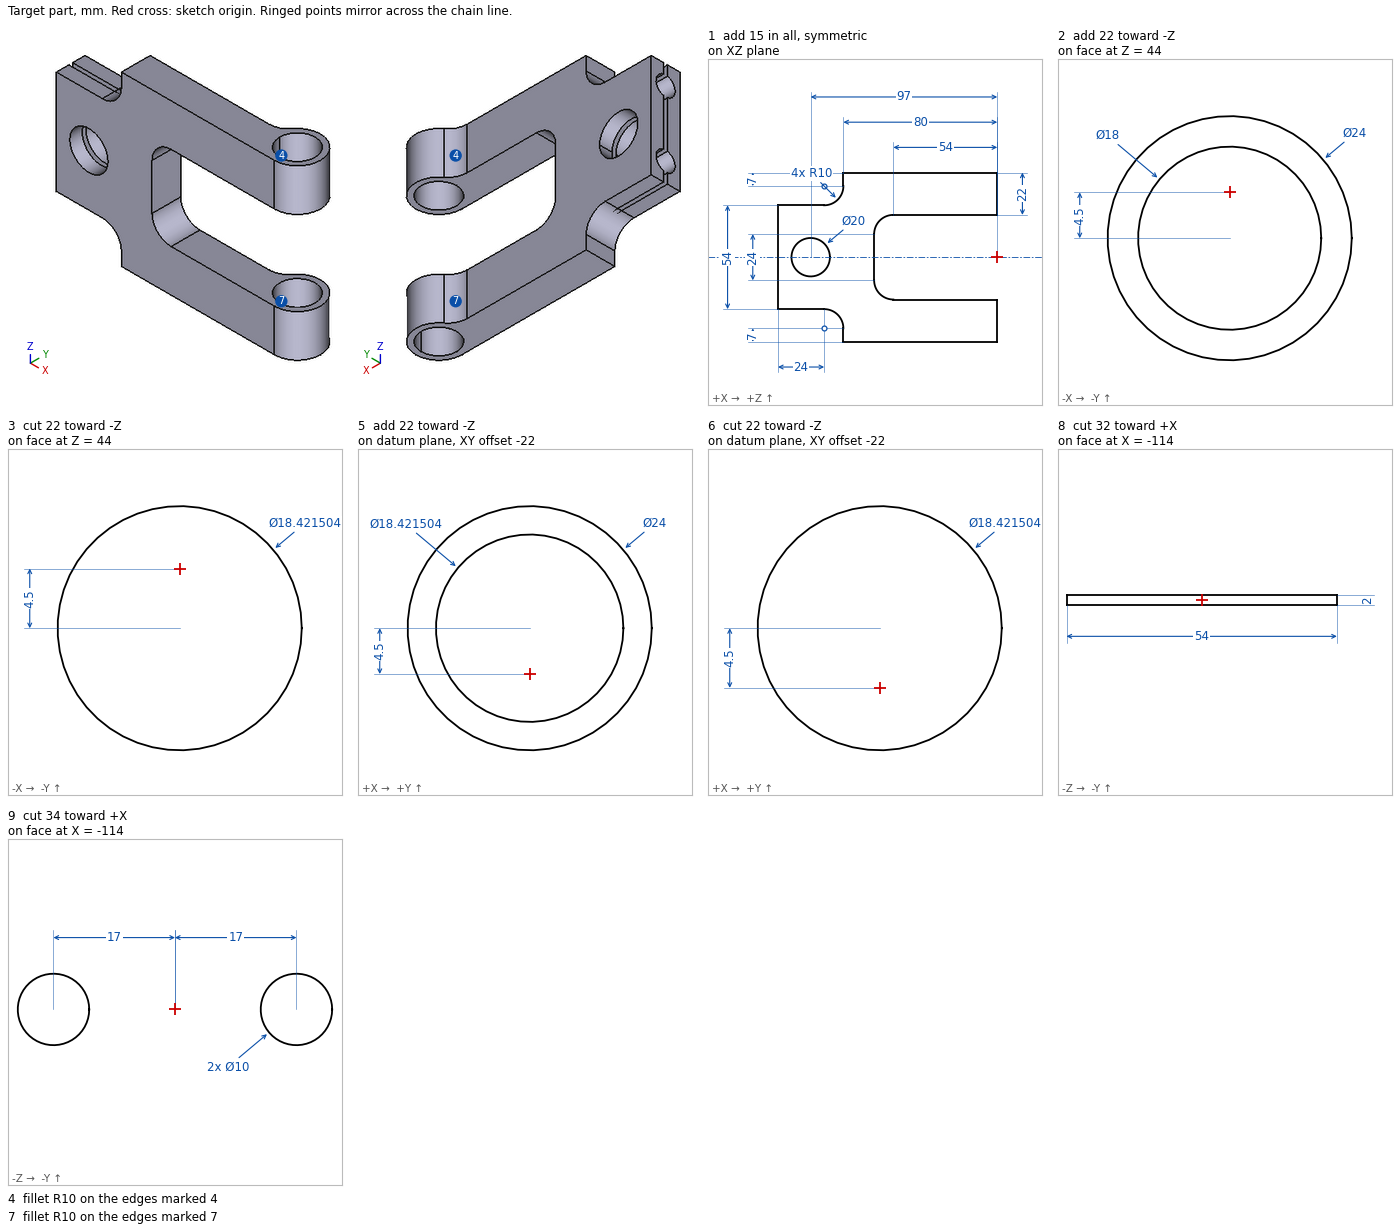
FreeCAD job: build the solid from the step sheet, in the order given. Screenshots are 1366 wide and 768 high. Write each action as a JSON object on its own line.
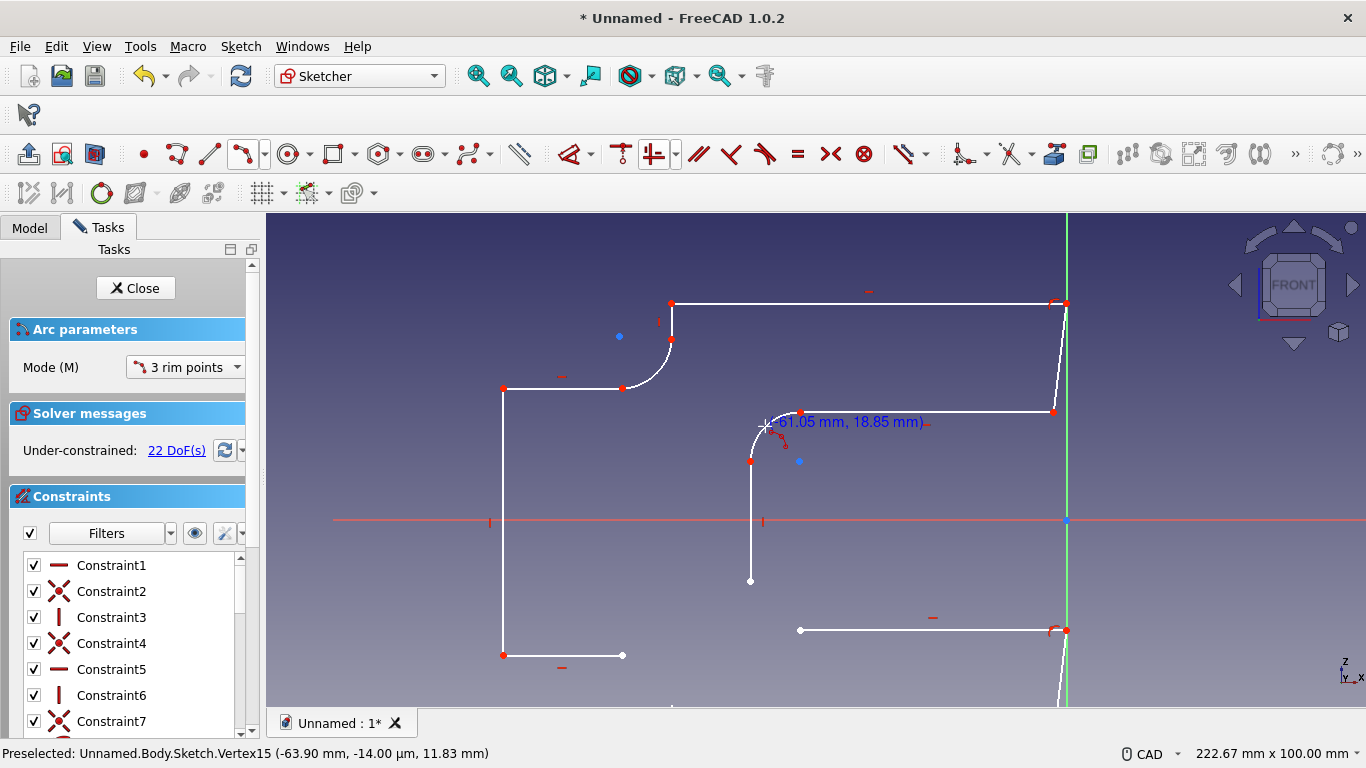
{"action": "left_click", "coordinate": [751, 581]}
{"action": "left_click", "coordinate": [800, 630]}
{"action": "left_click", "coordinate": [765, 614]}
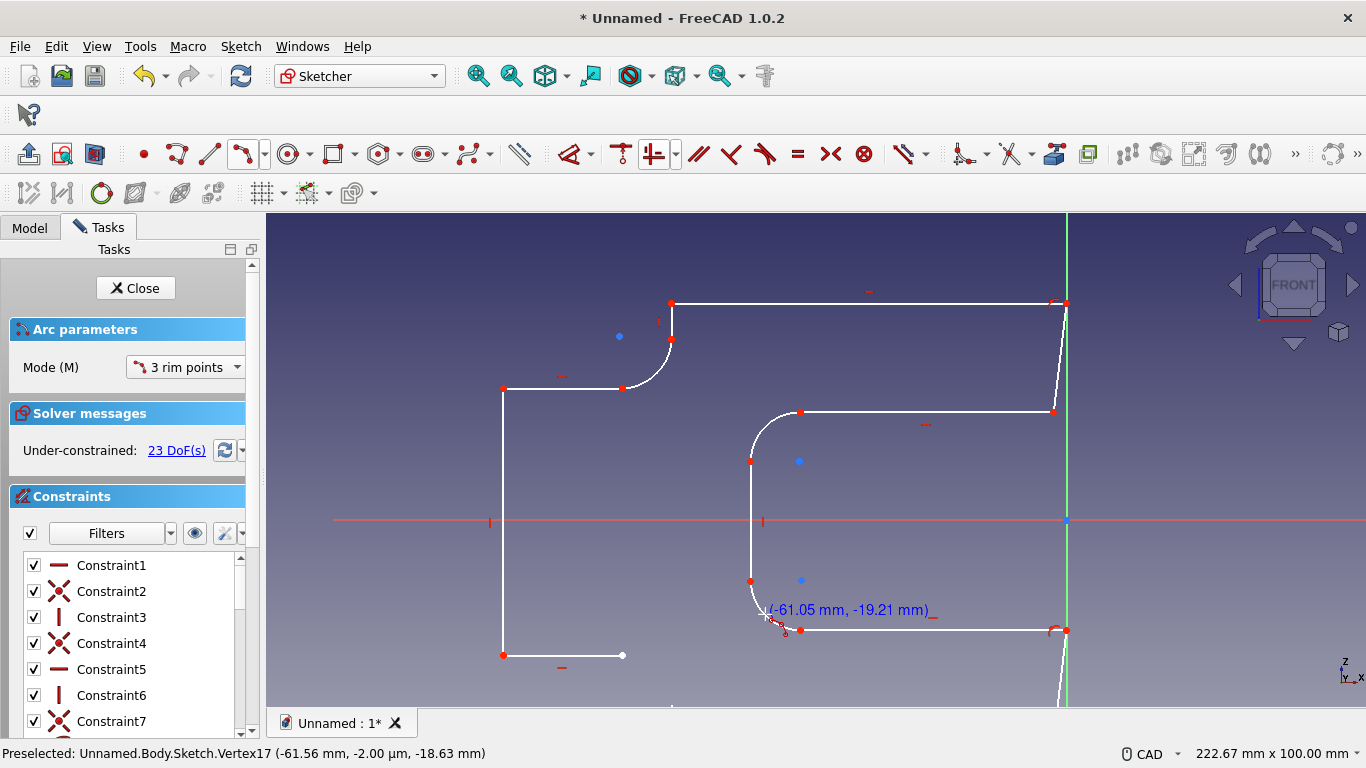
{"action": "scroll", "coordinate": [671, 338], "scroll_direction": "down", "scroll_amount": 2}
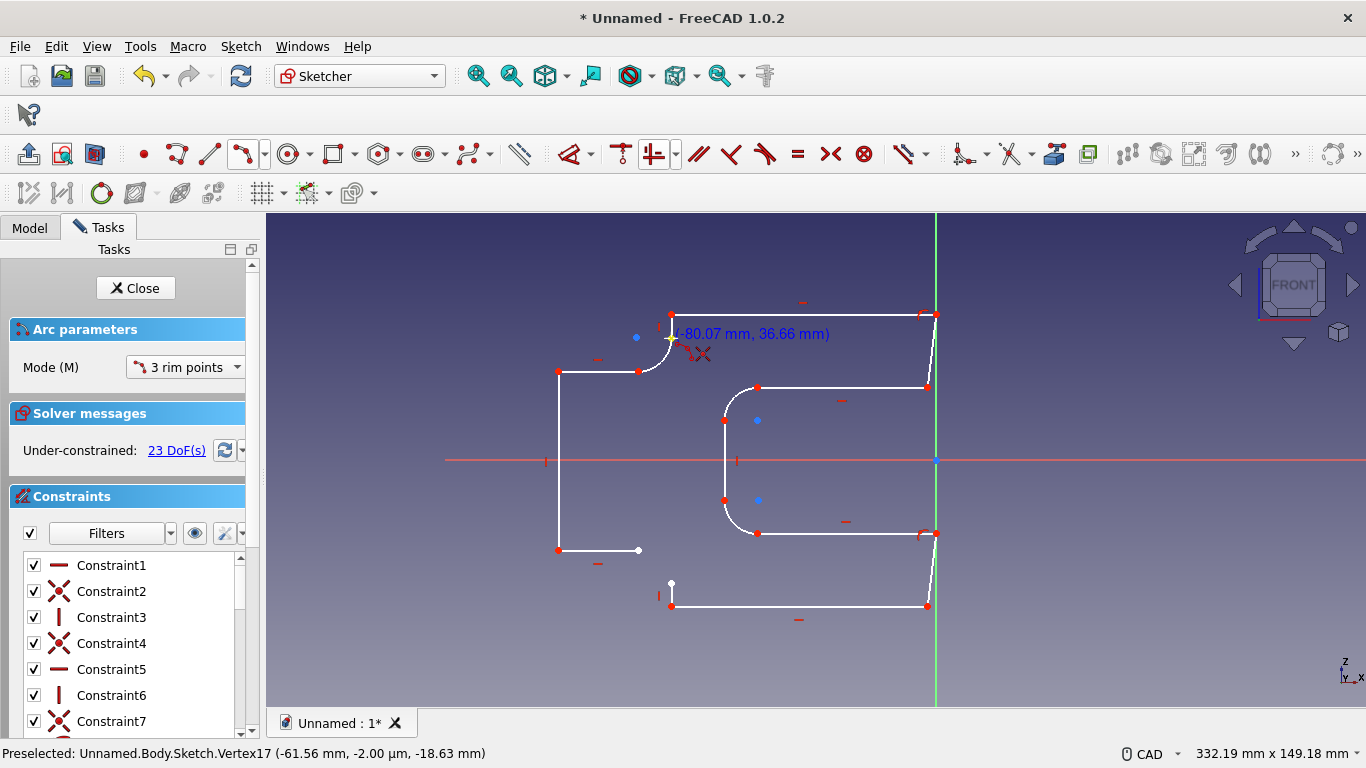
{"action": "scroll", "coordinate": [671, 583], "scroll_direction": "up", "scroll_amount": 2}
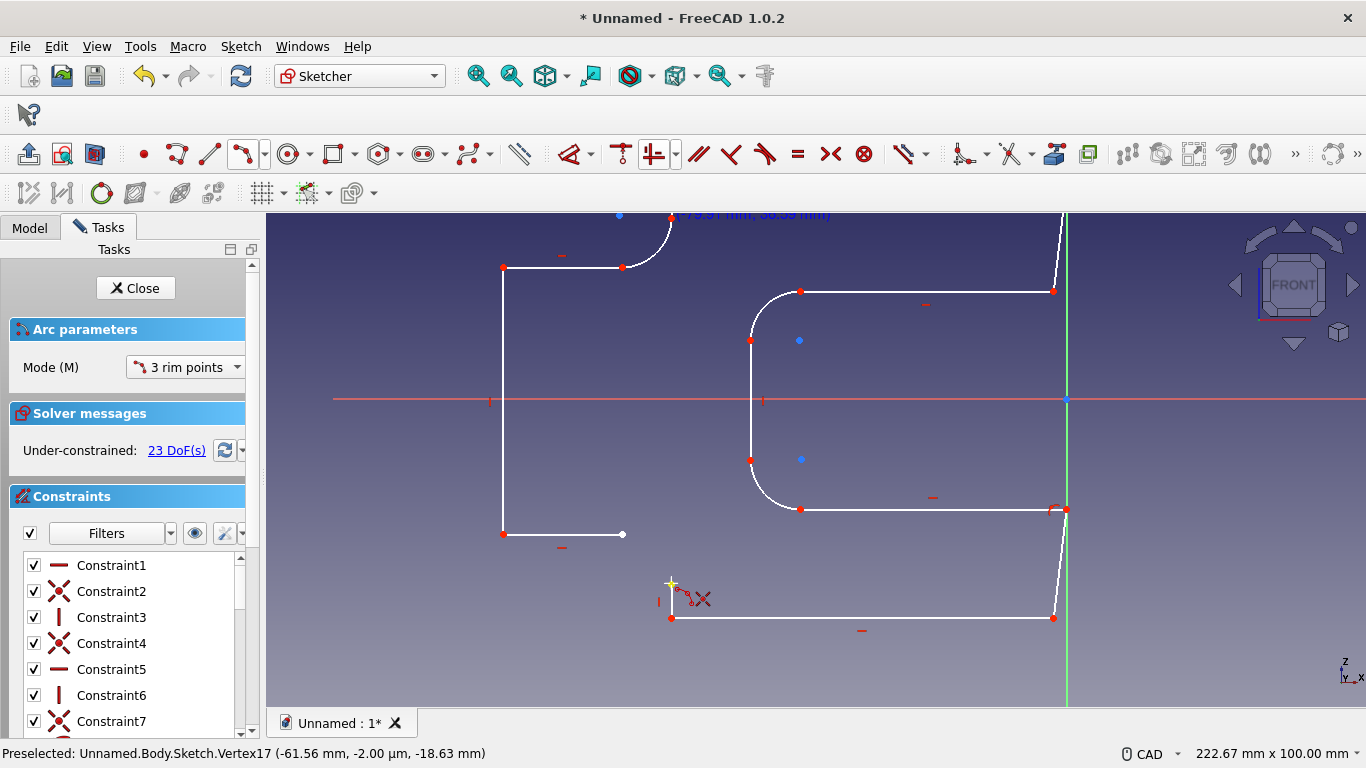
{"action": "left_click", "coordinate": [672, 584]}
{"action": "left_click", "coordinate": [623, 535]}
{"action": "left_click", "coordinate": [657, 547]}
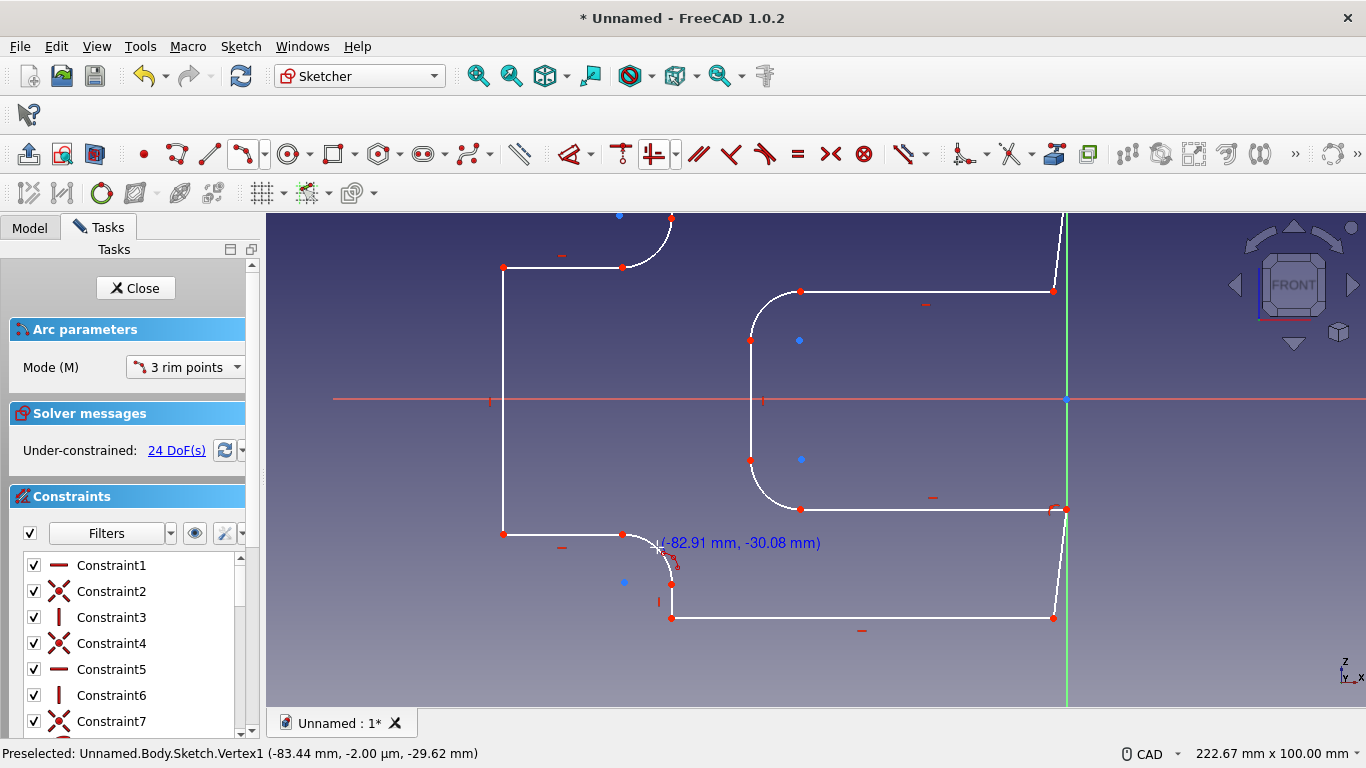
{"action": "left_click", "coordinate": [288, 154]}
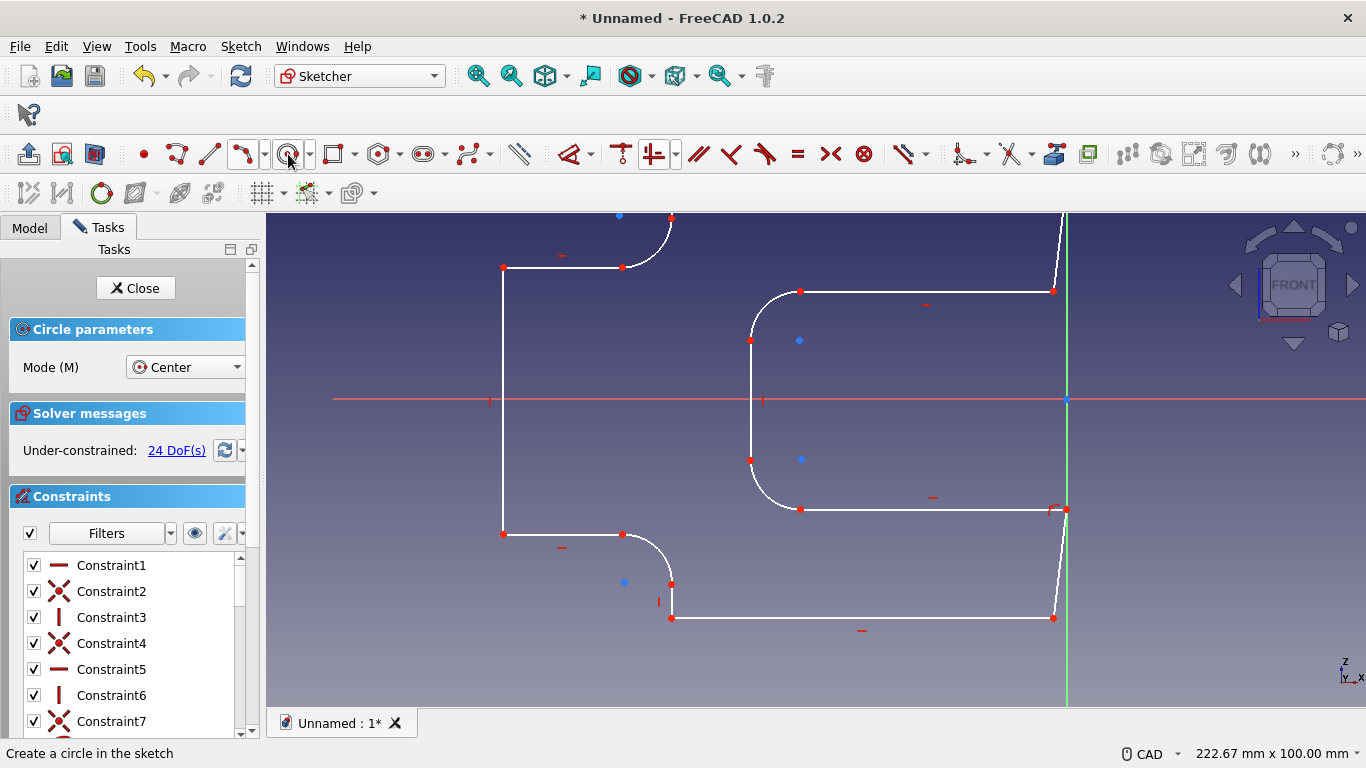
{"action": "left_click", "coordinate": [587, 399]}
{"action": "left_click", "coordinate": [622, 364]}
{"action": "key", "text": "Escape"}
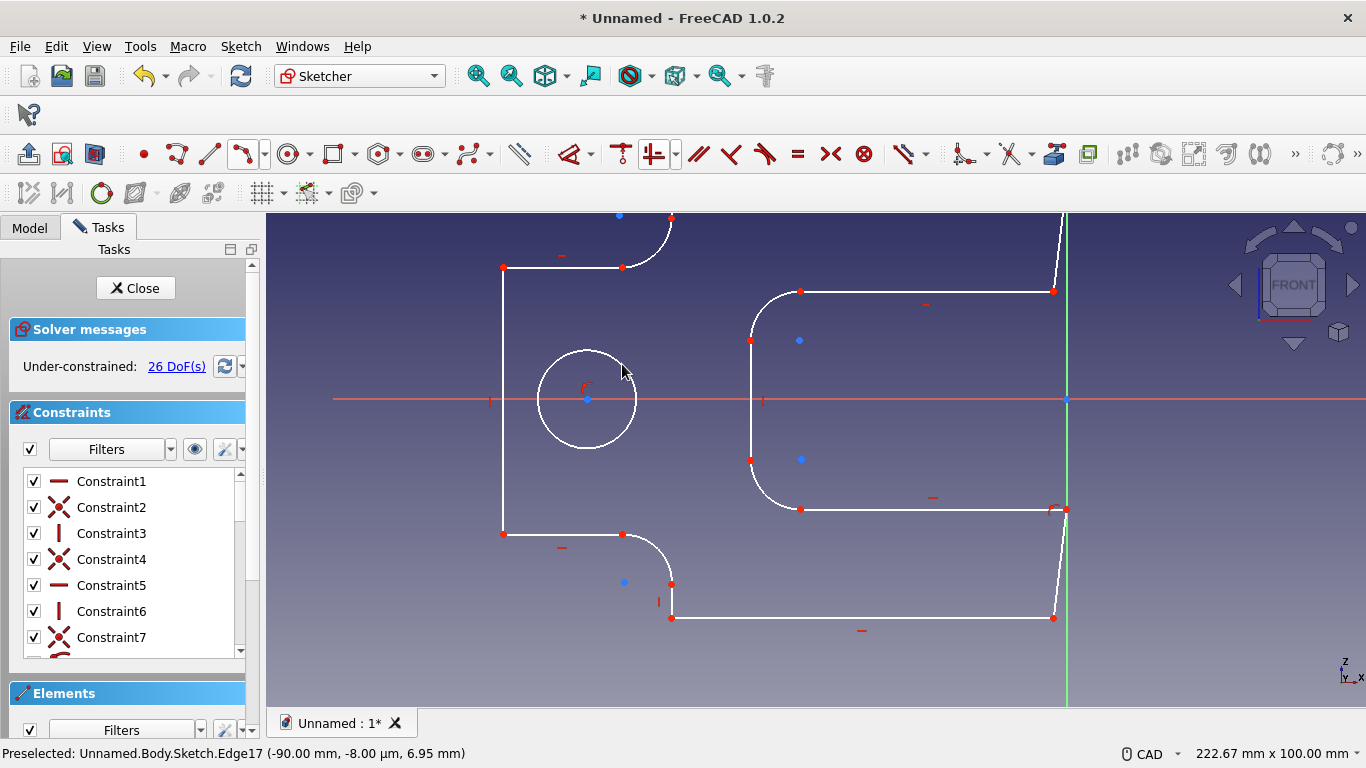
{"action": "left_click", "coordinate": [587, 535]}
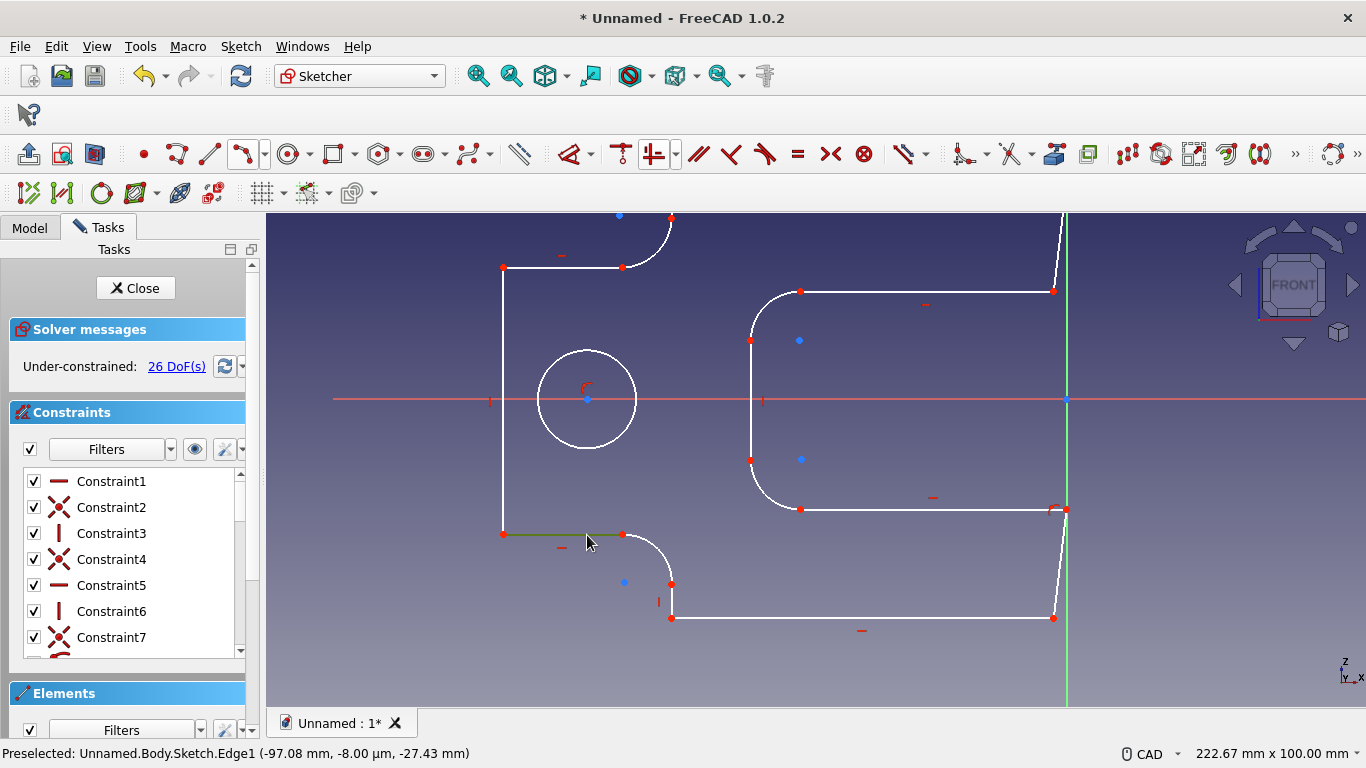
{"action": "left_click", "coordinate": [667, 561]}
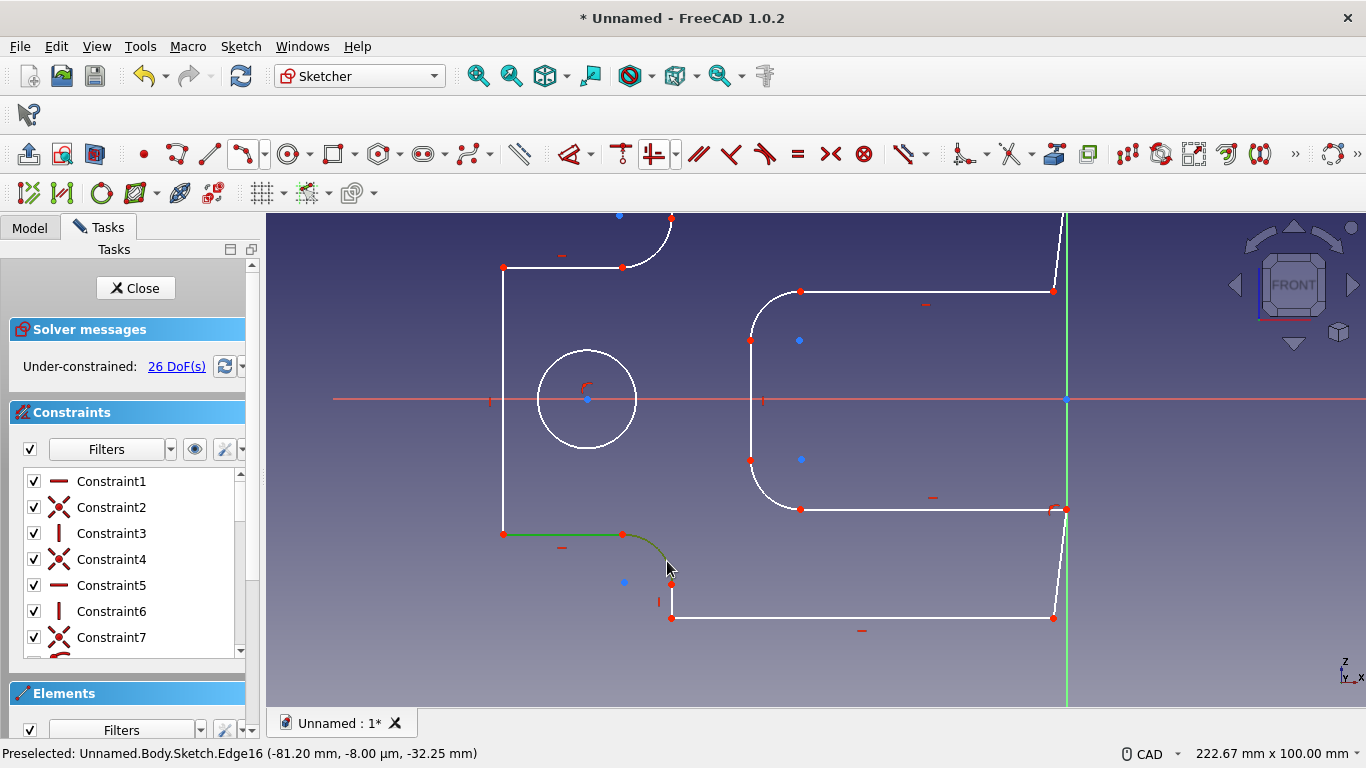
{"action": "left_click", "coordinate": [765, 154]}